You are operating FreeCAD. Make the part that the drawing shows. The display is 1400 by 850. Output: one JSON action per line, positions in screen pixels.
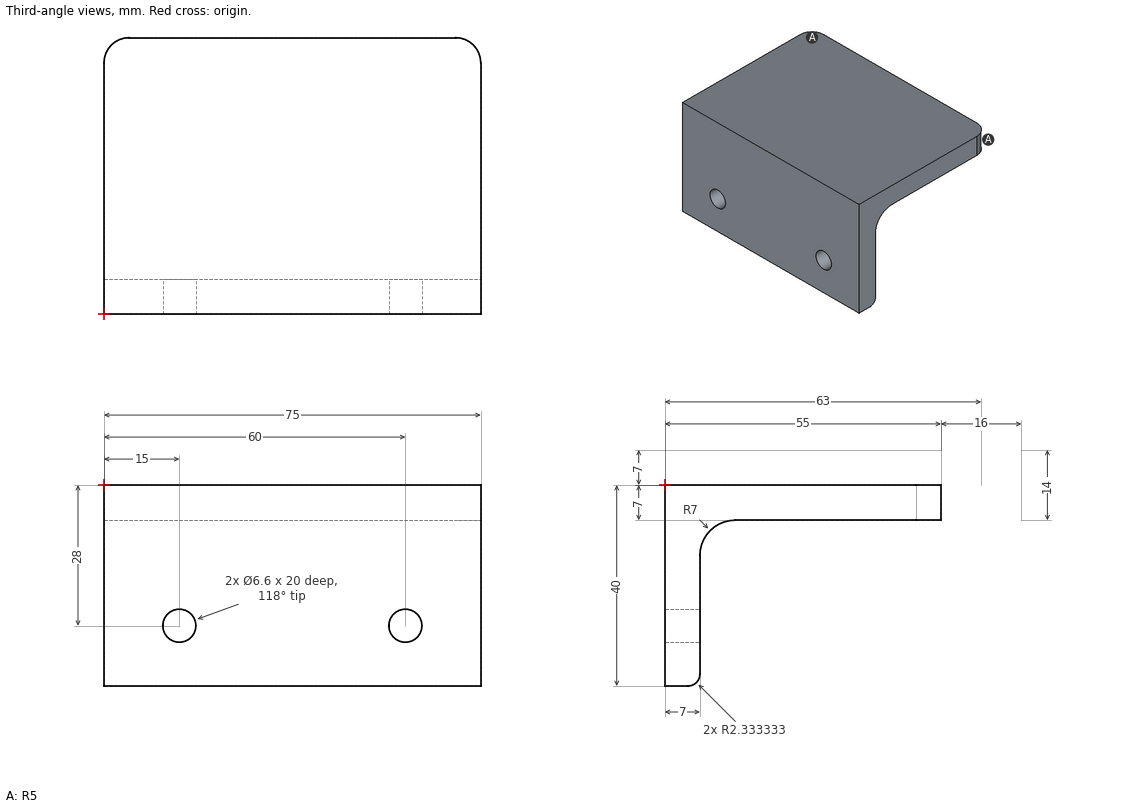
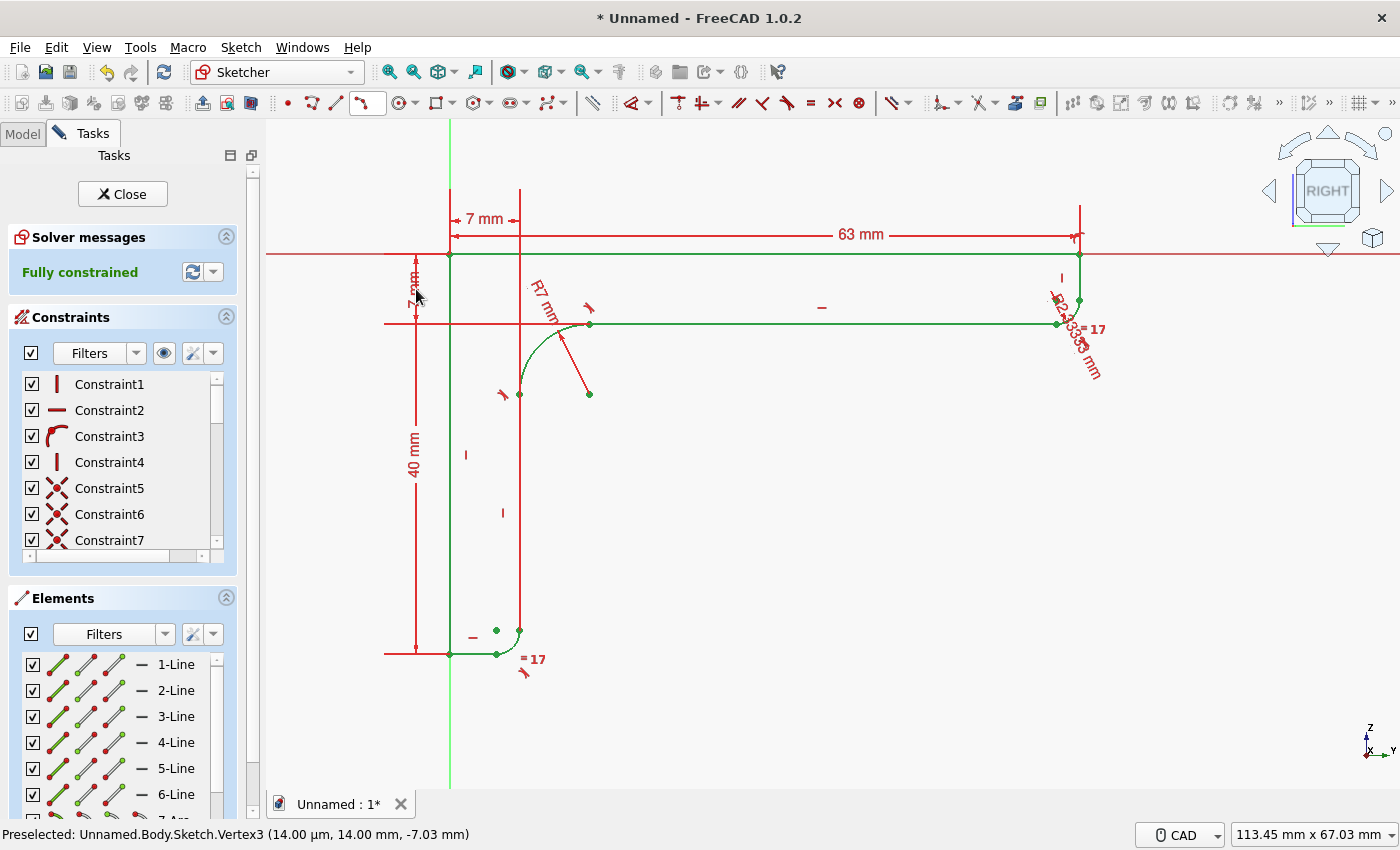
{"action": "left_click", "coordinate": [123, 194]}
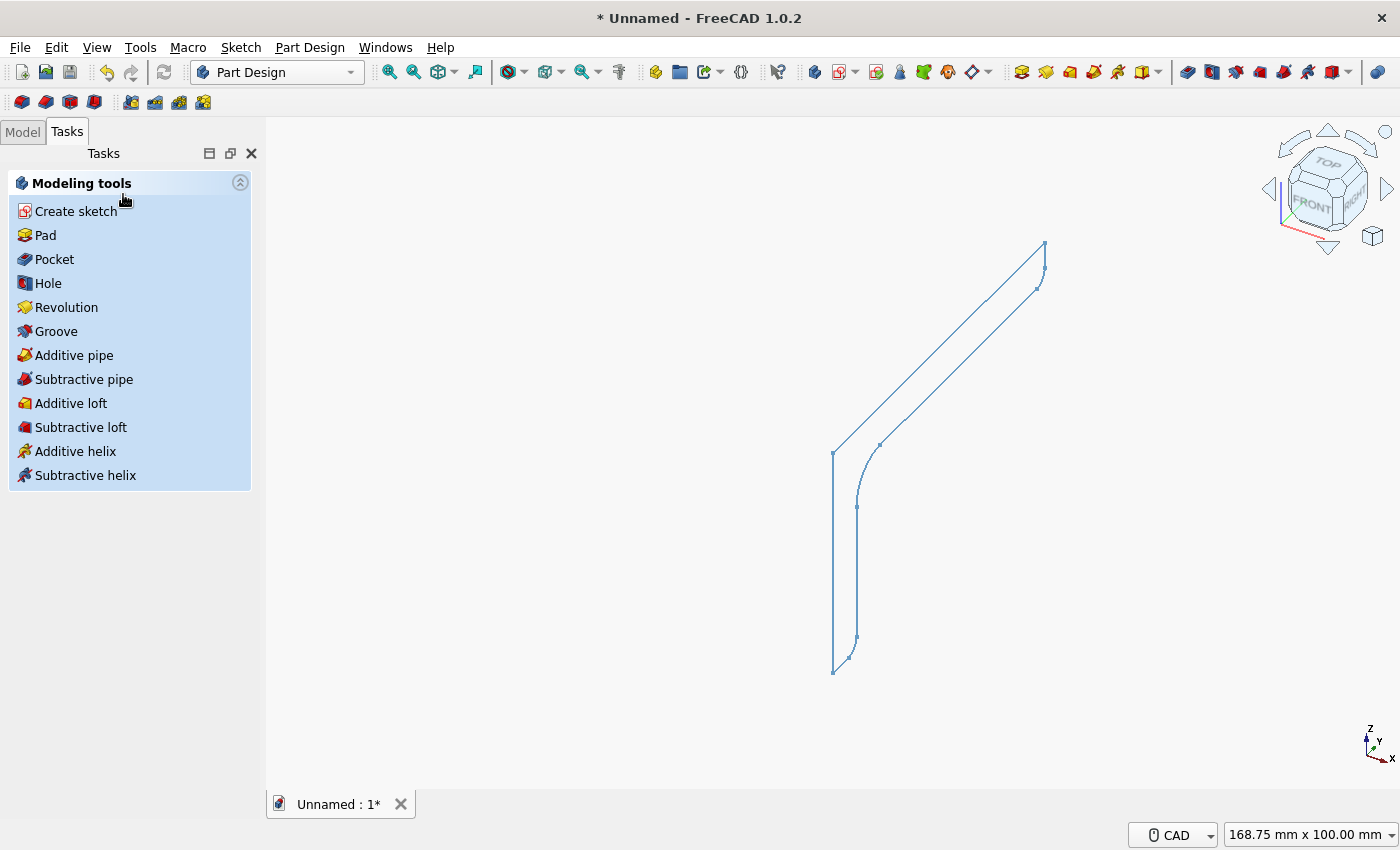
{"action": "left_click", "coordinate": [1022, 72]}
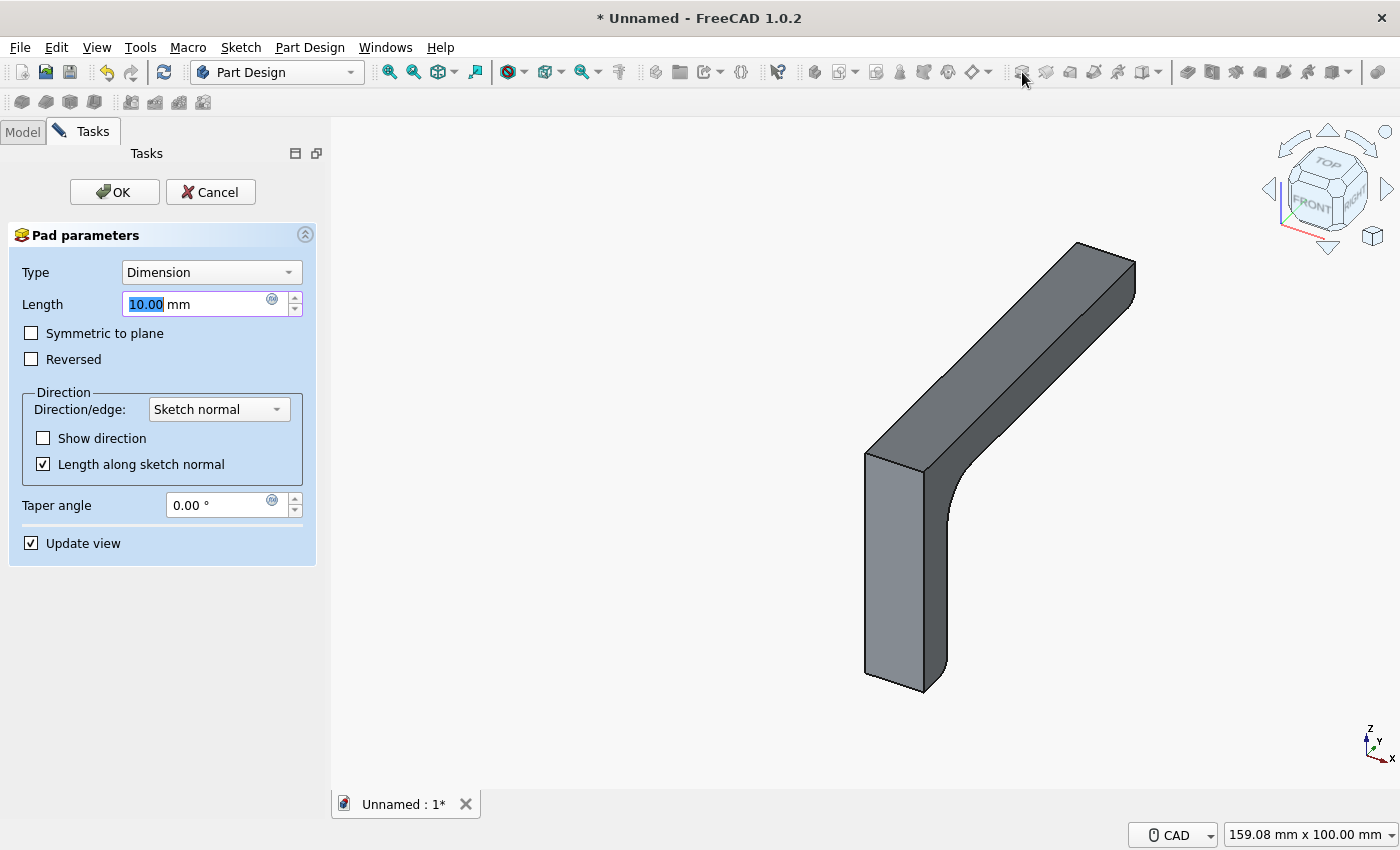
{"action": "type", "text": "75"}
{"action": "key", "text": "Tab"}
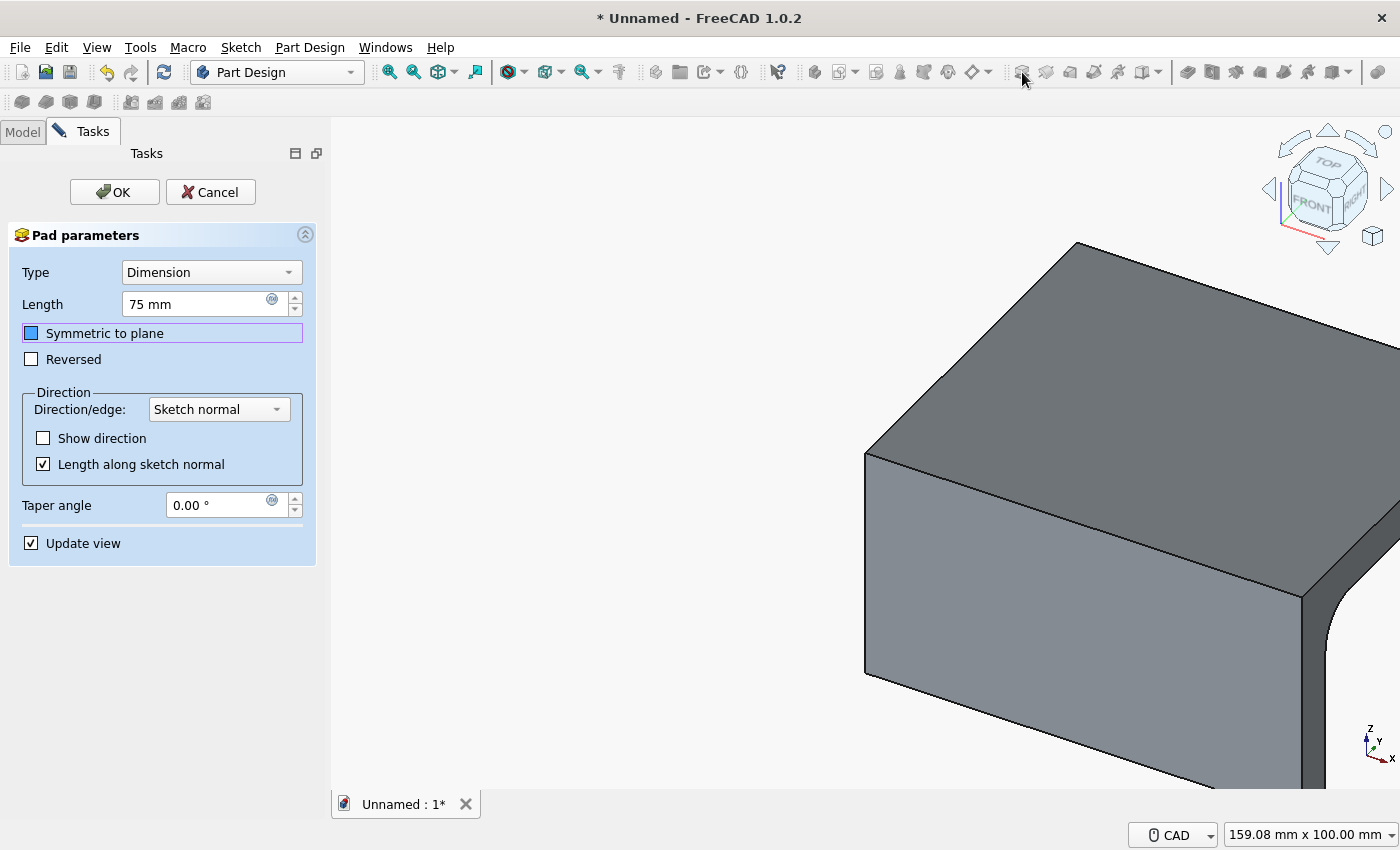
{"action": "left_click", "coordinate": [115, 192]}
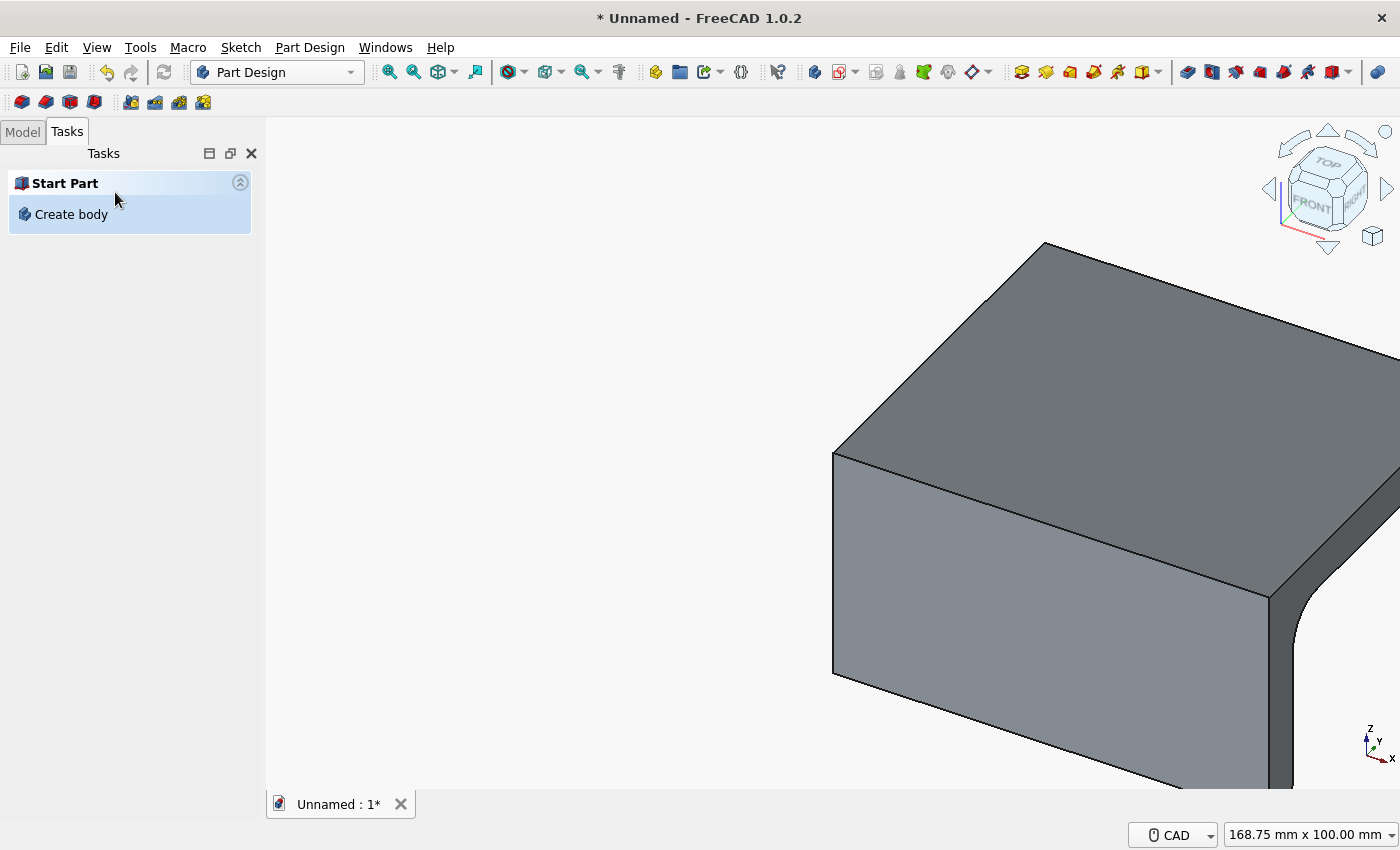
{"action": "left_click", "coordinate": [390, 72]}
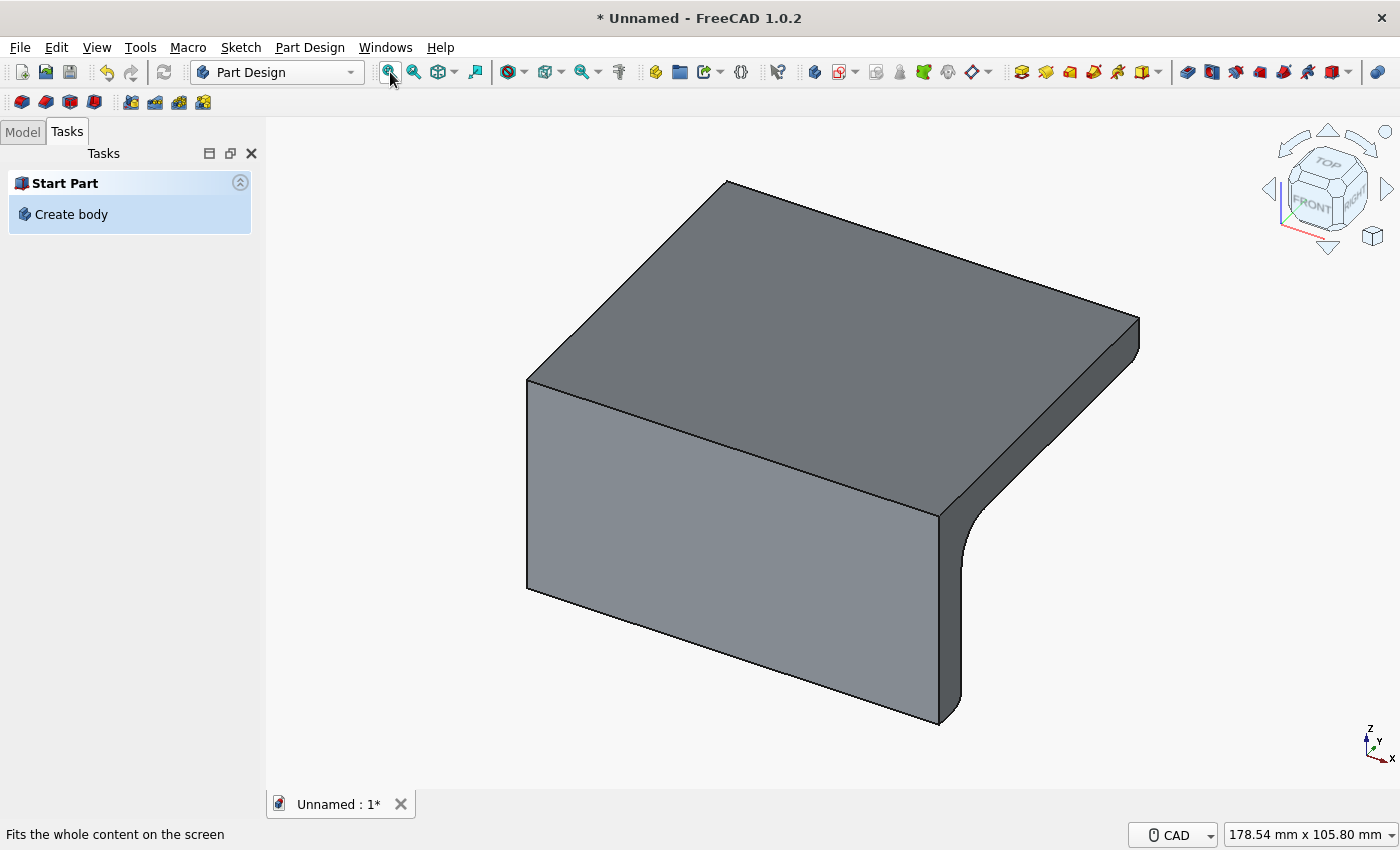
{"action": "left_click", "coordinate": [840, 72]}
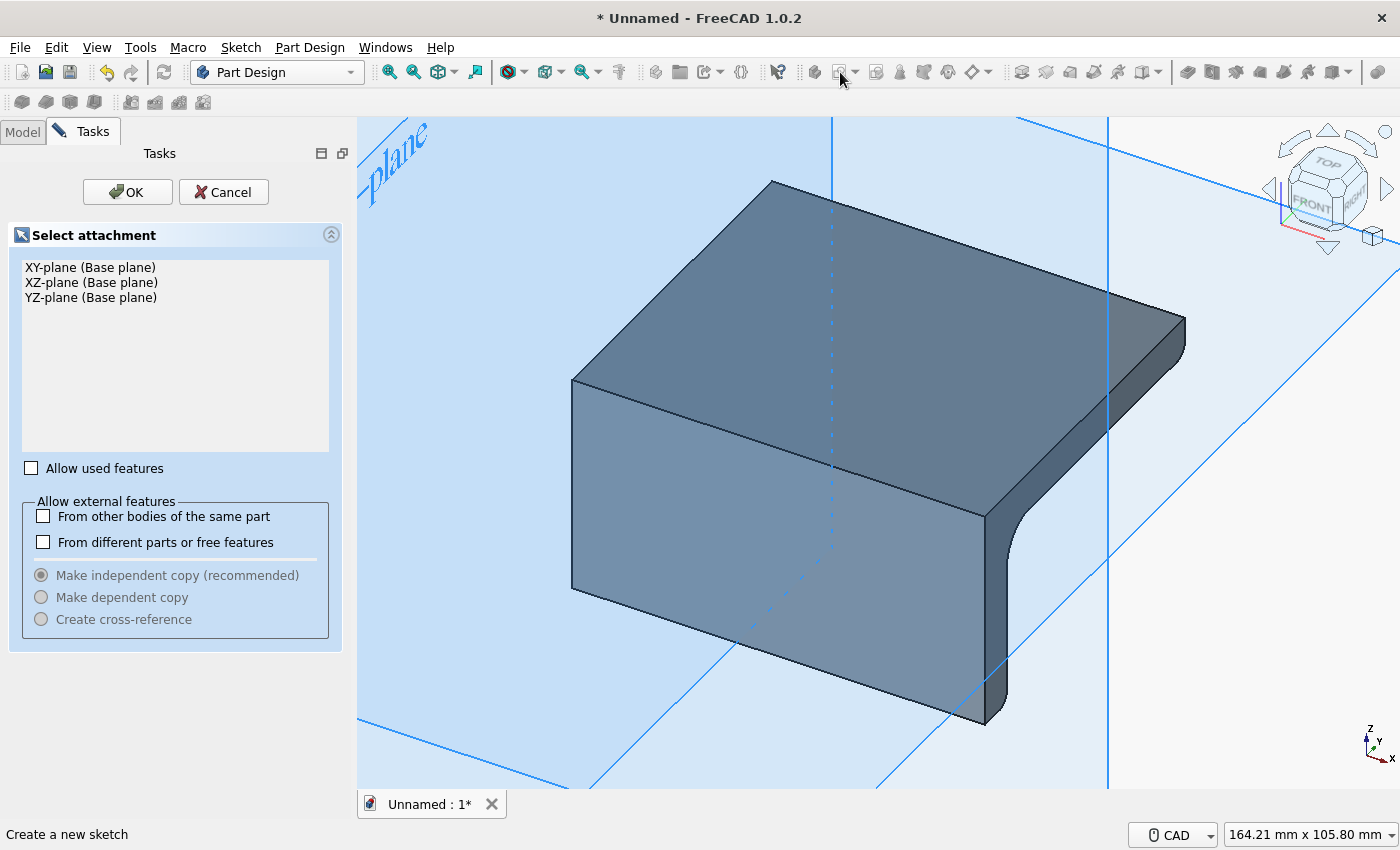
{"action": "left_click", "coordinate": [82, 282]}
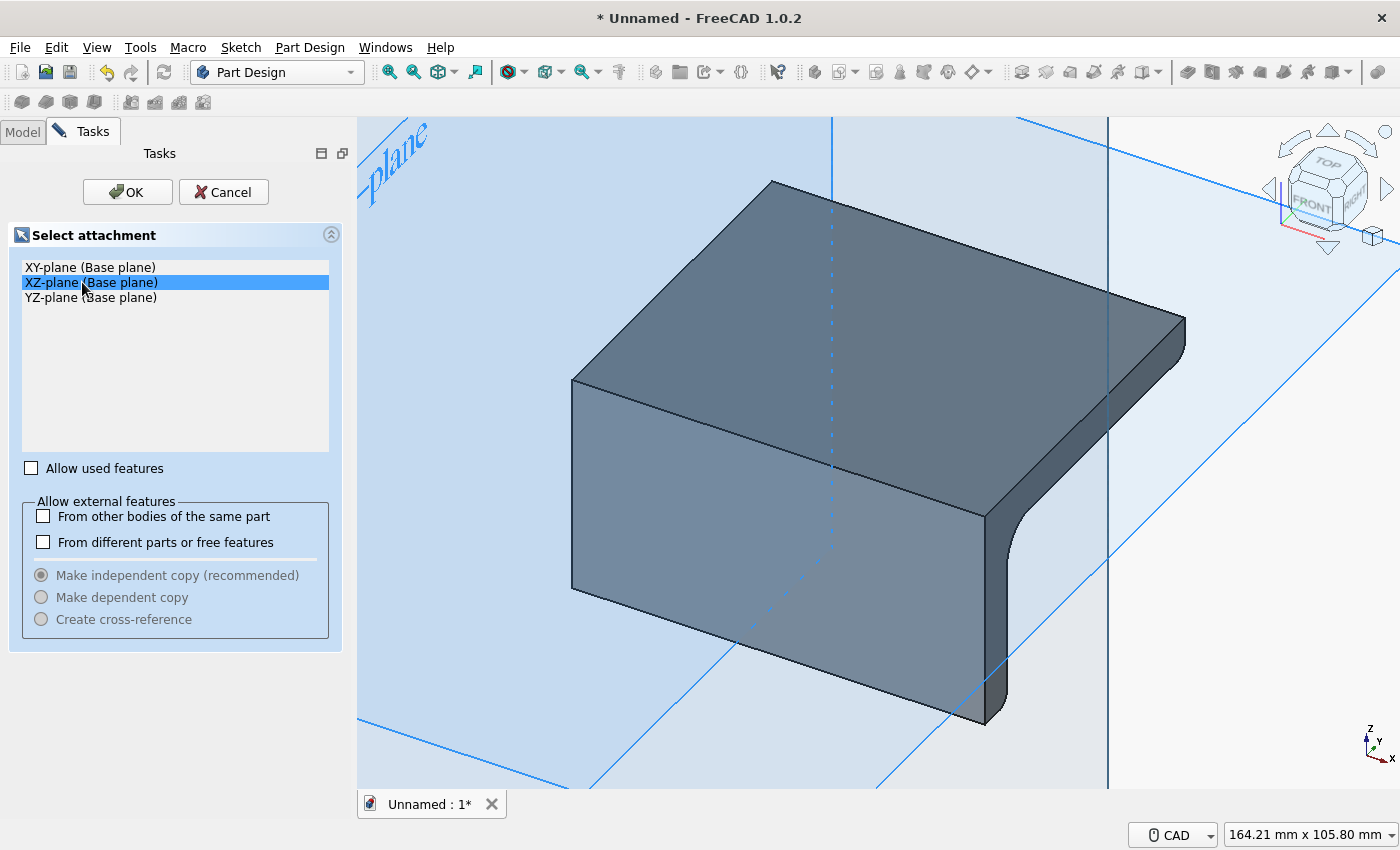
{"action": "left_click", "coordinate": [128, 192]}